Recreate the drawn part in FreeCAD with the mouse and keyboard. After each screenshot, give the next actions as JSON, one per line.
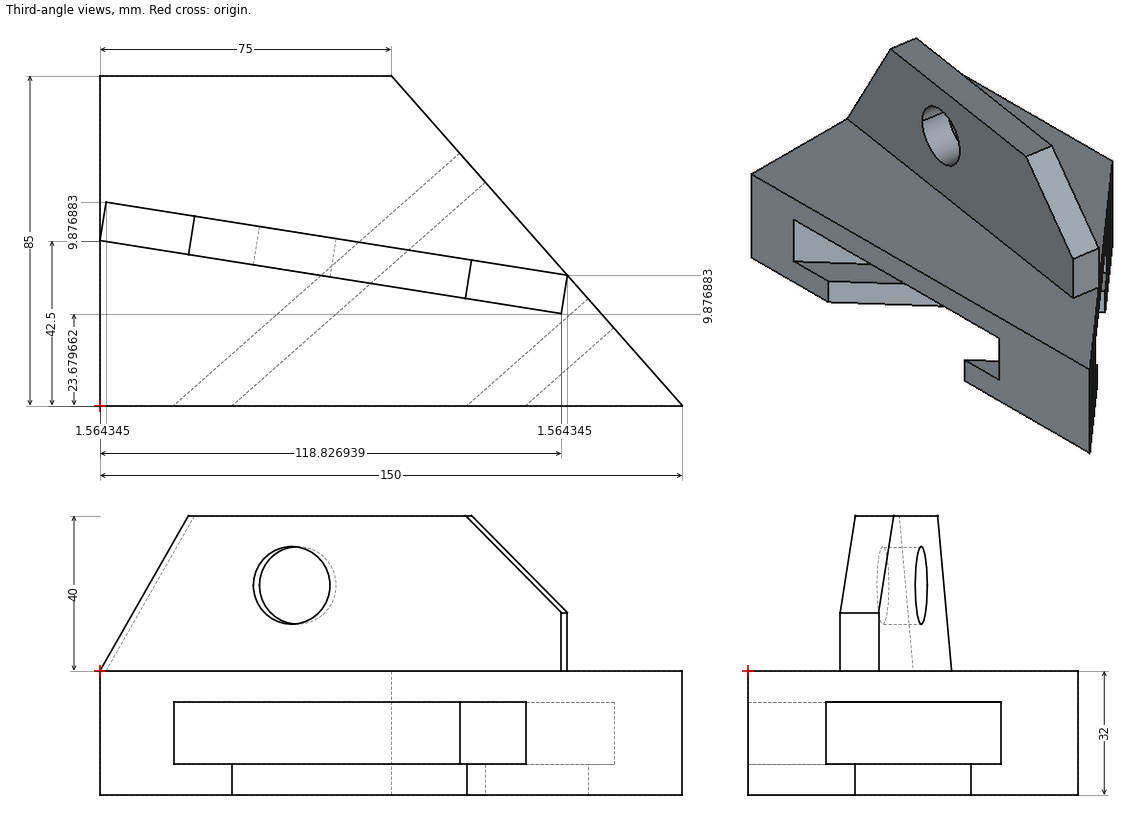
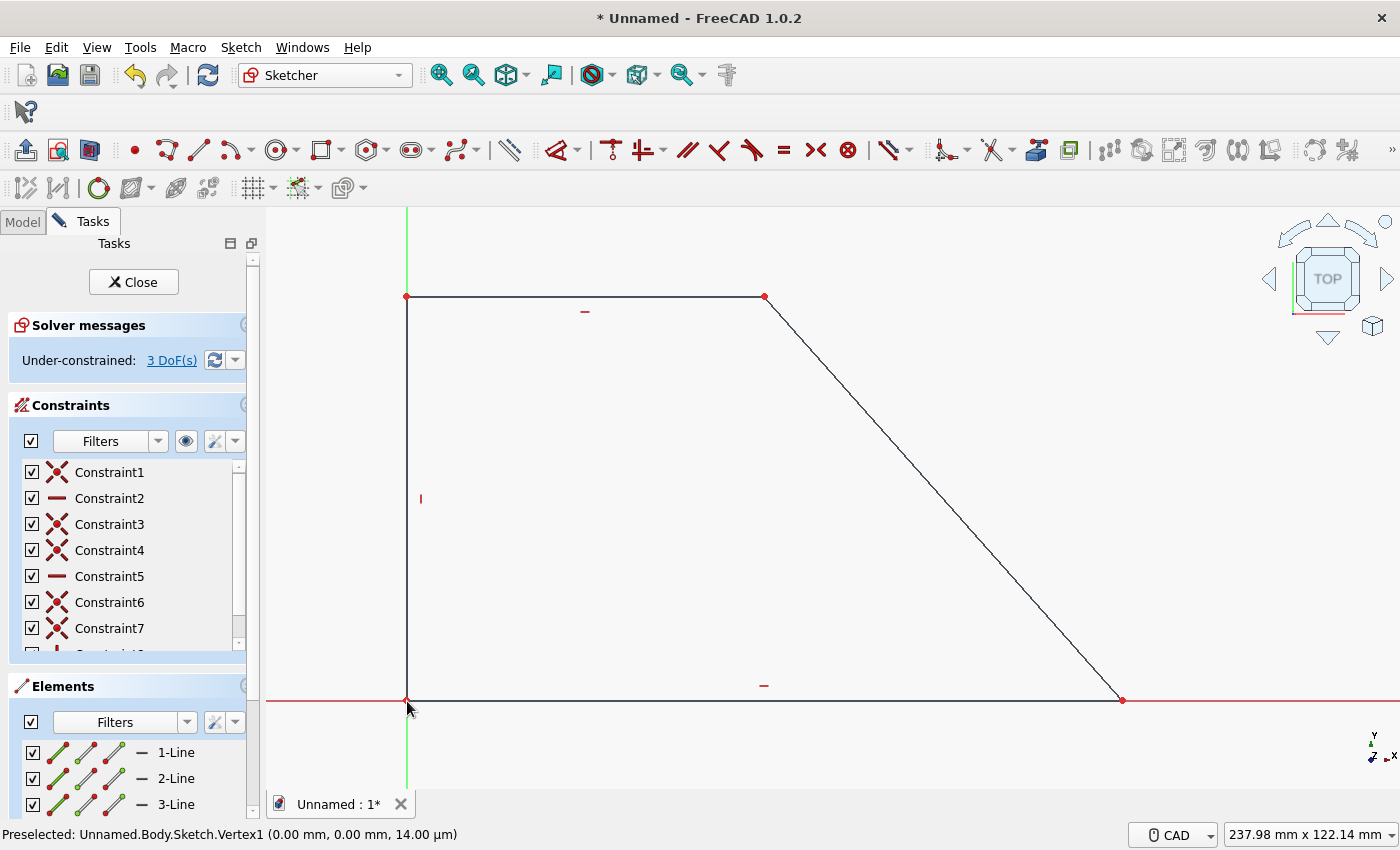
{"action": "left_click", "coordinate": [657, 297]}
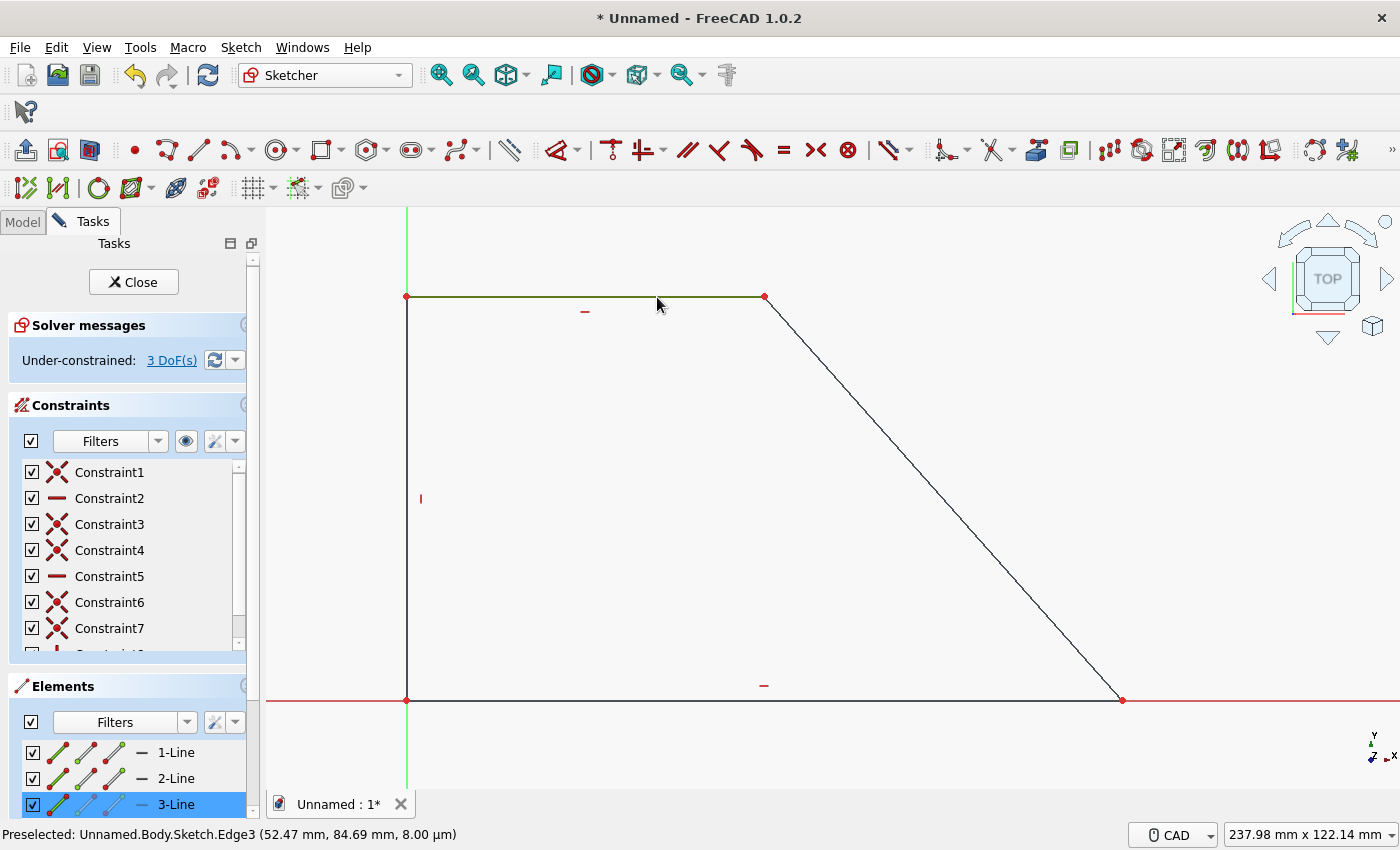
{"action": "key", "text": "l"}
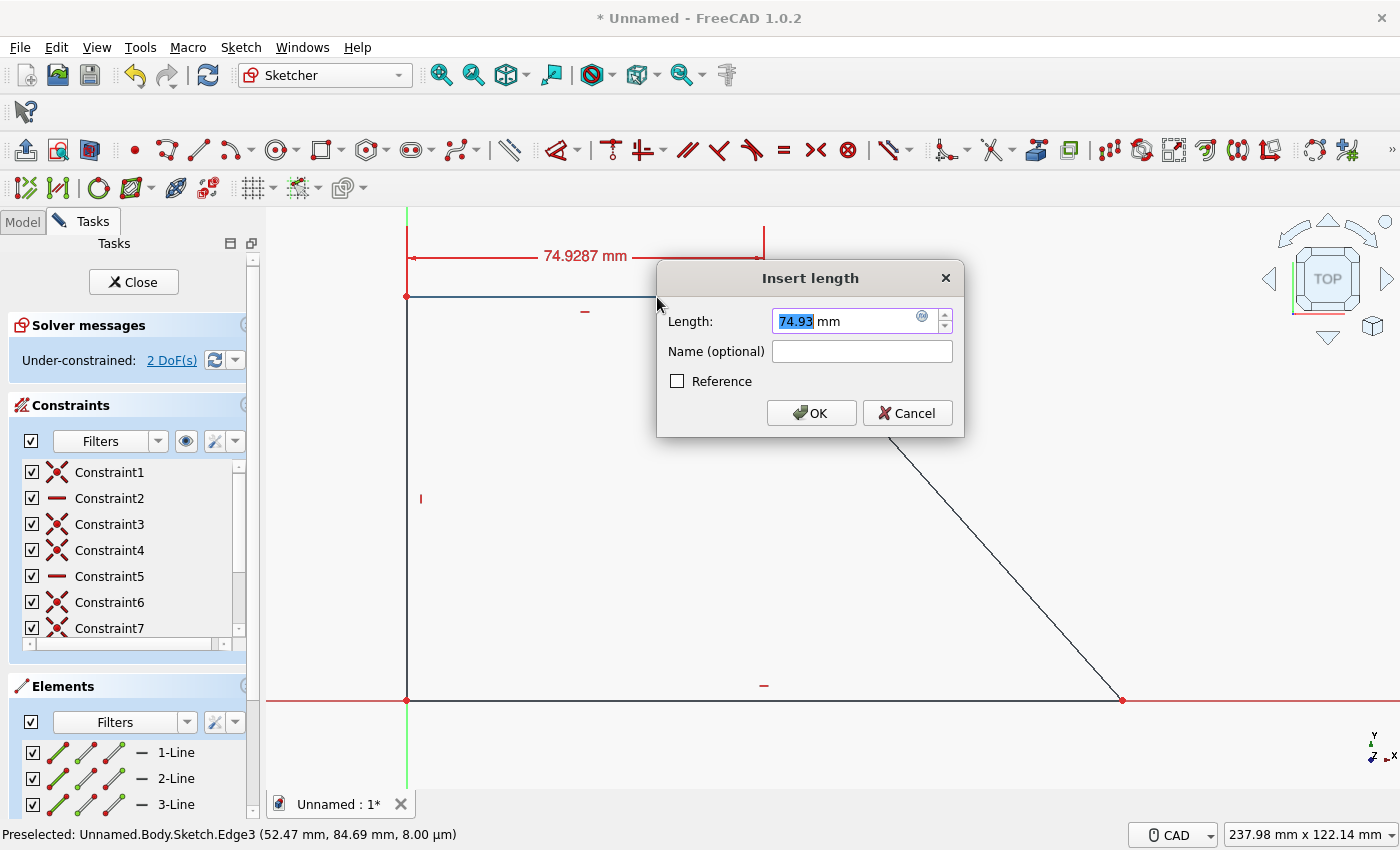
{"action": "type", "text": "75"}
{"action": "key", "text": "Return"}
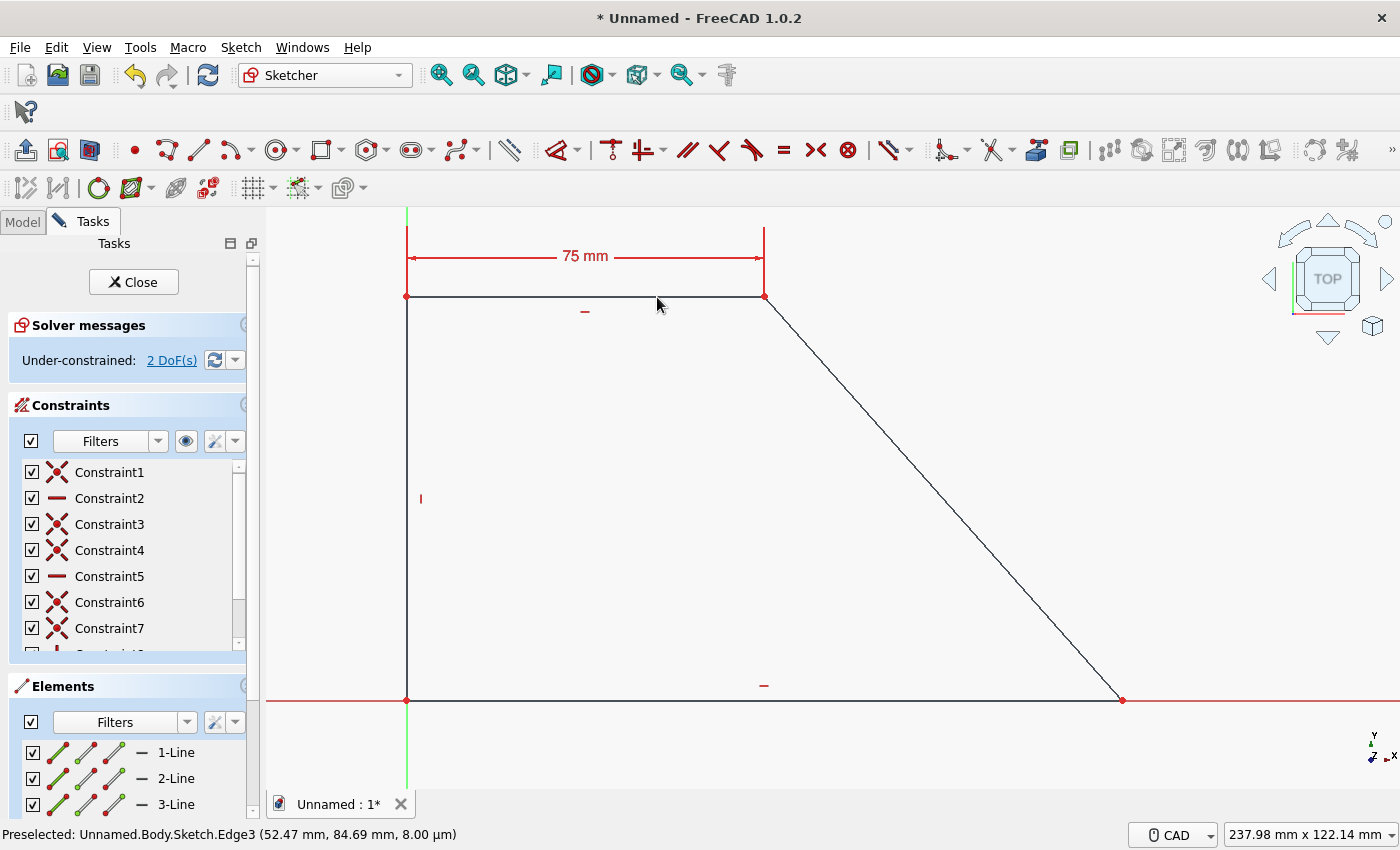
{"action": "left_click", "coordinate": [407, 418]}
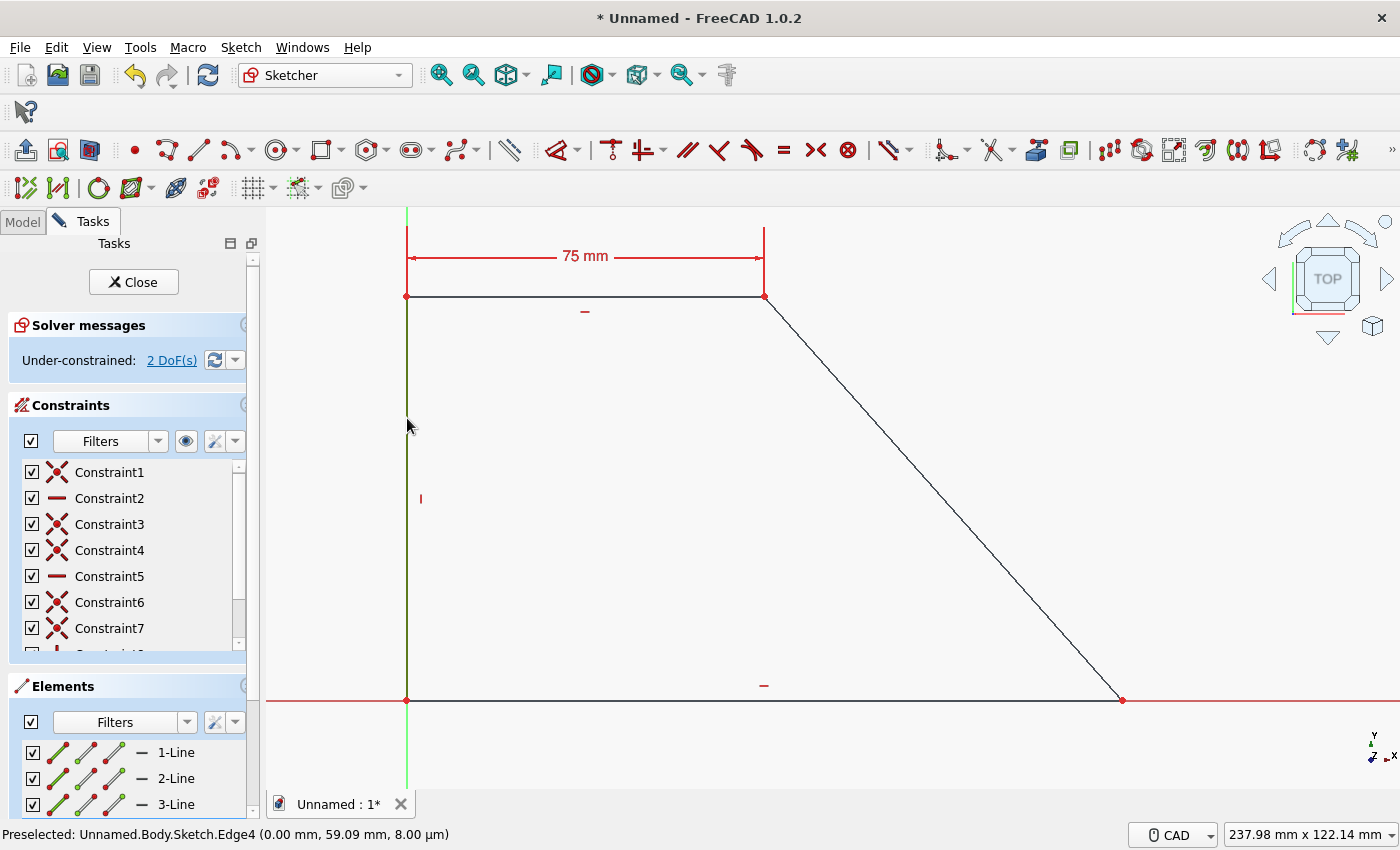
{"action": "key", "text": "i"}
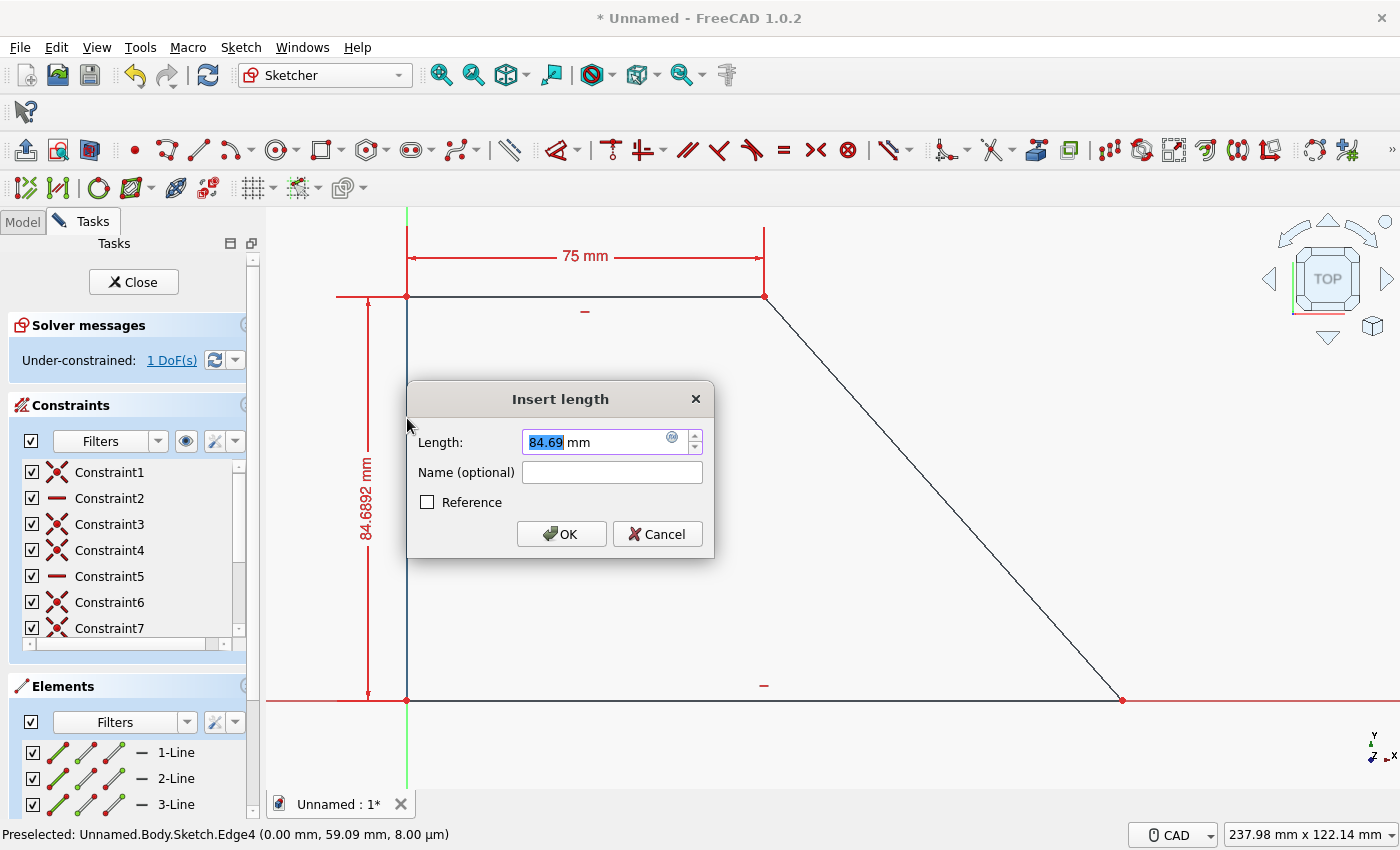
{"action": "type", "text": "85"}
{"action": "key", "text": "Return"}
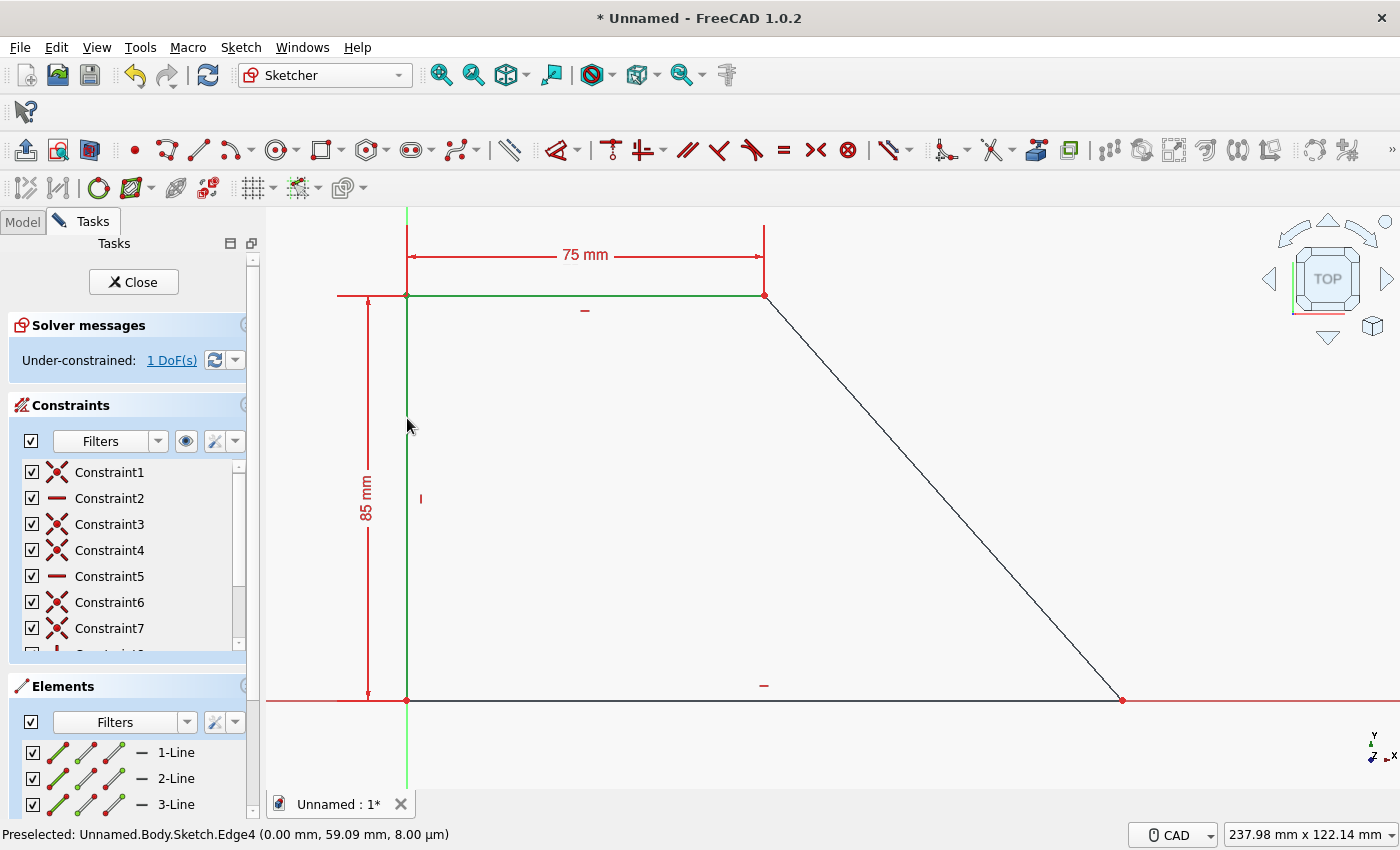
{"action": "left_click", "coordinate": [621, 701]}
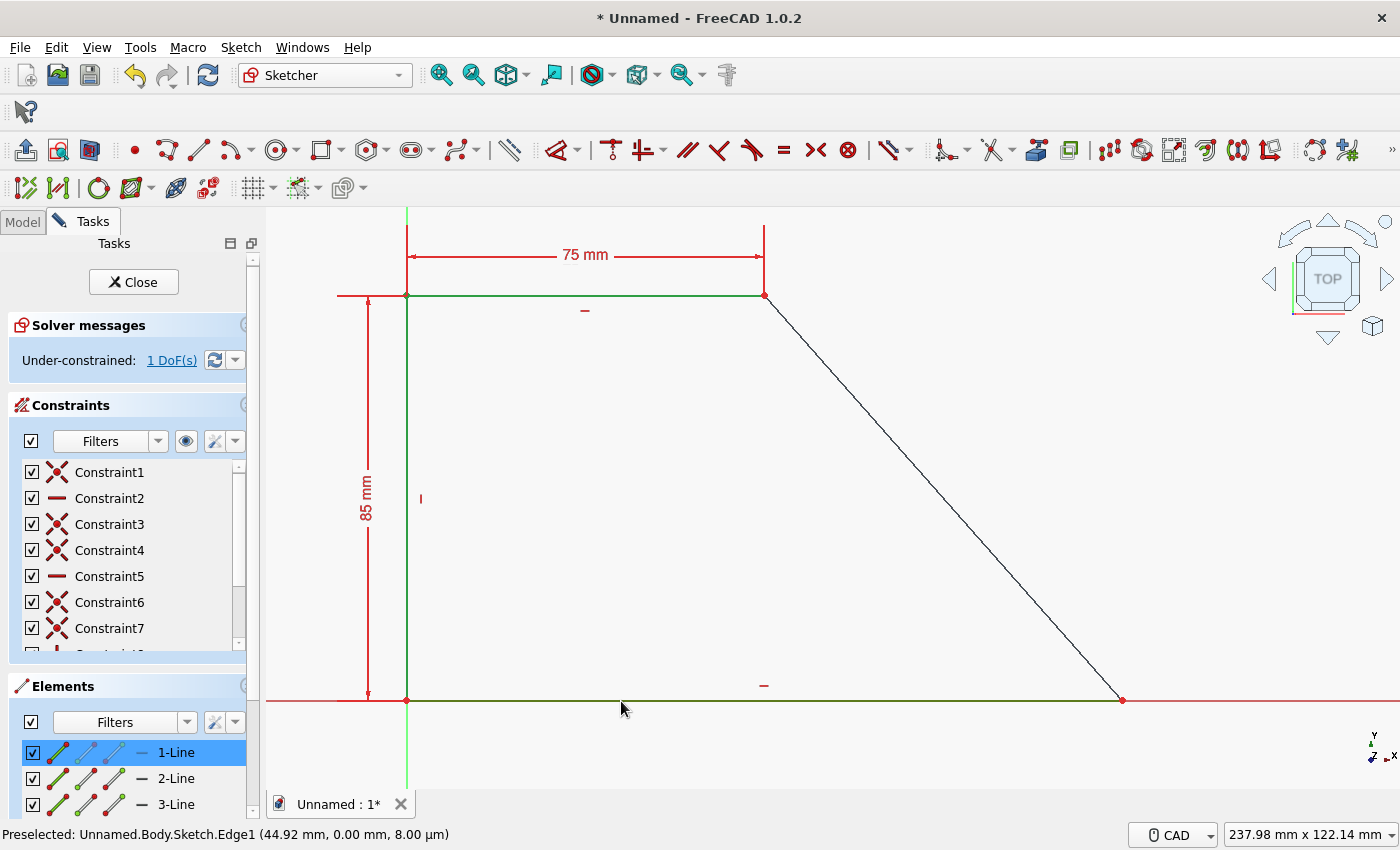
{"action": "left_click", "coordinate": [580, 150]}